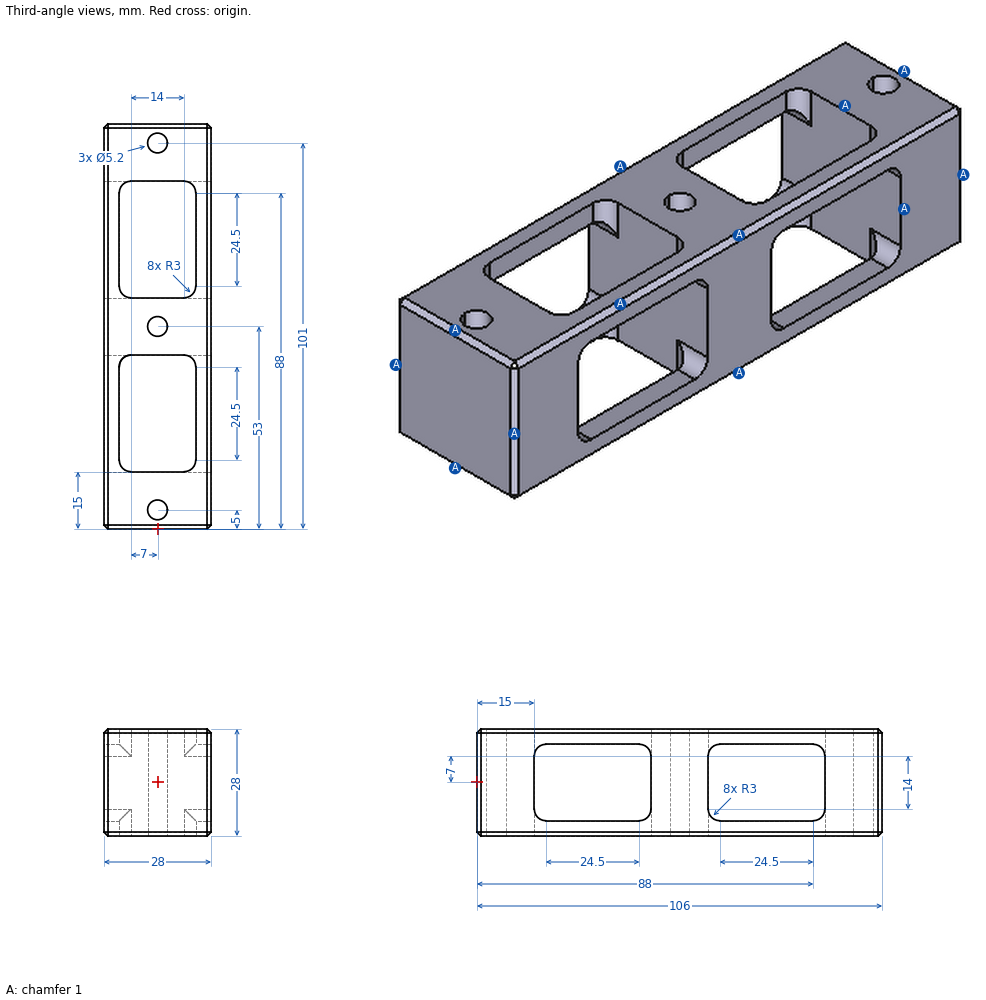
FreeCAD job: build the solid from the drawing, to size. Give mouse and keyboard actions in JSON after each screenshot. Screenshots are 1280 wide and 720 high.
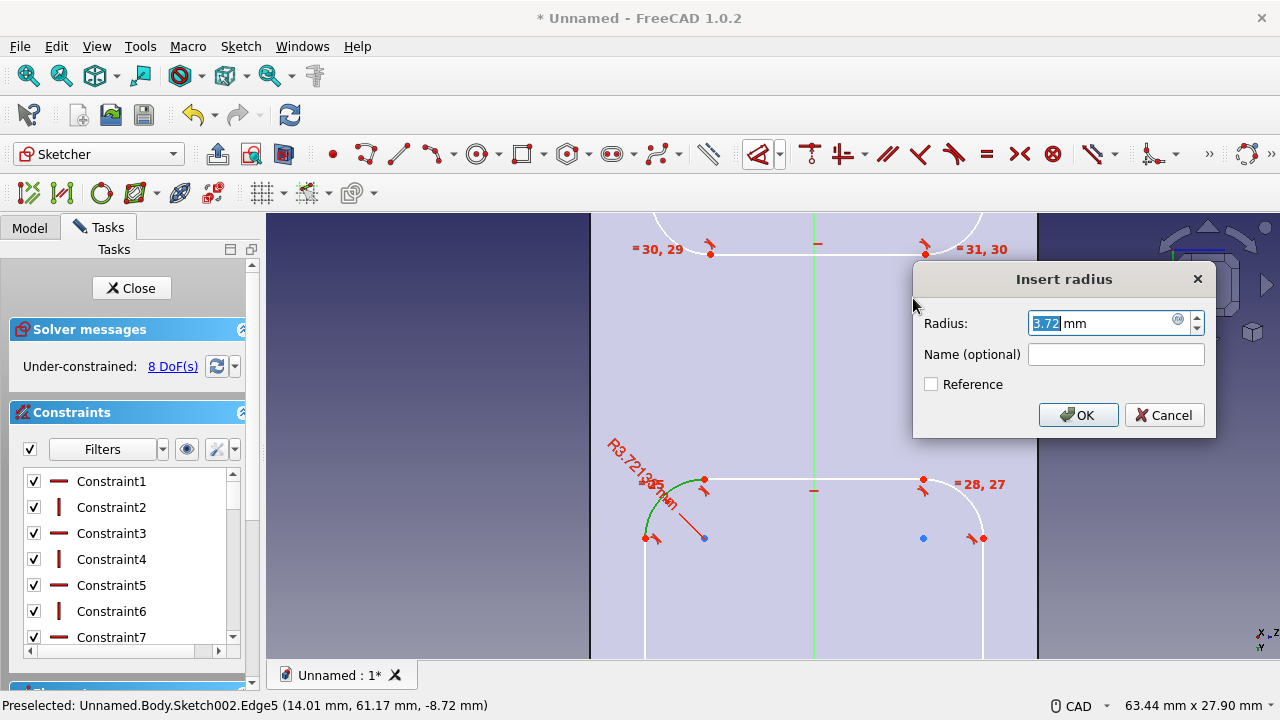
{"action": "type", "text": "3"}
{"action": "key", "text": "Return"}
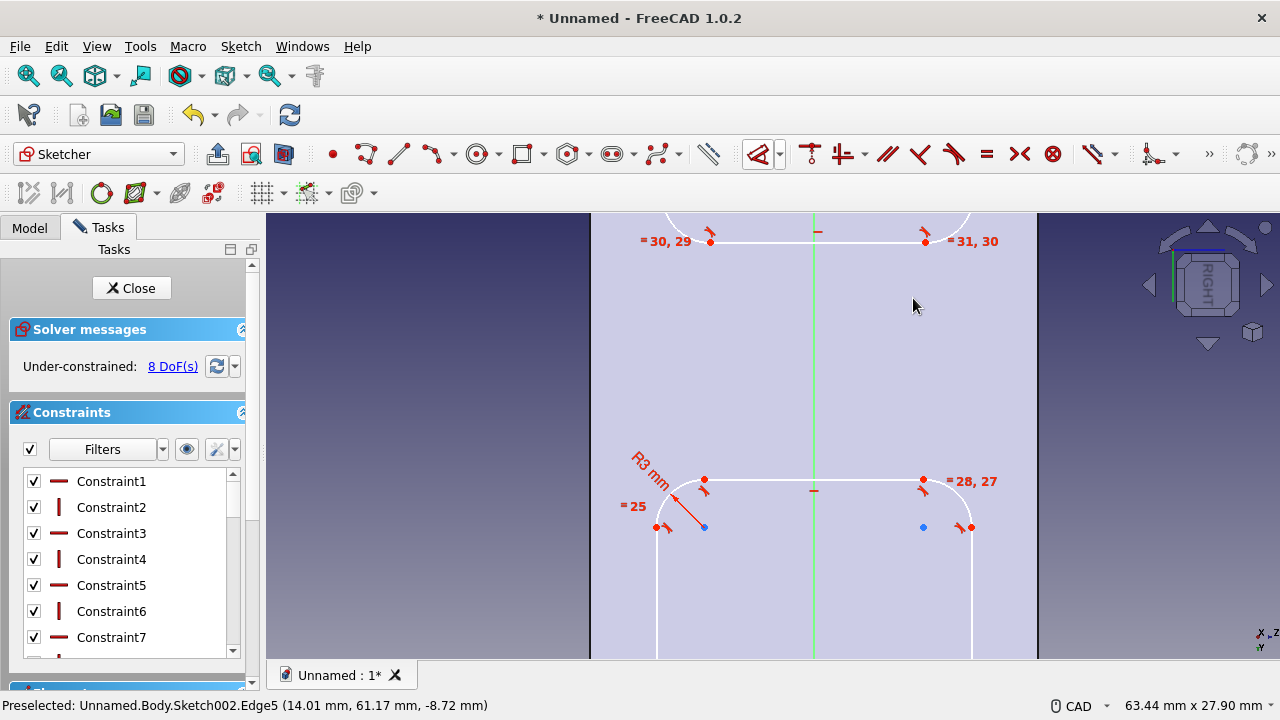
{"action": "scroll", "coordinate": [677, 486], "scroll_direction": "down", "scroll_amount": 8}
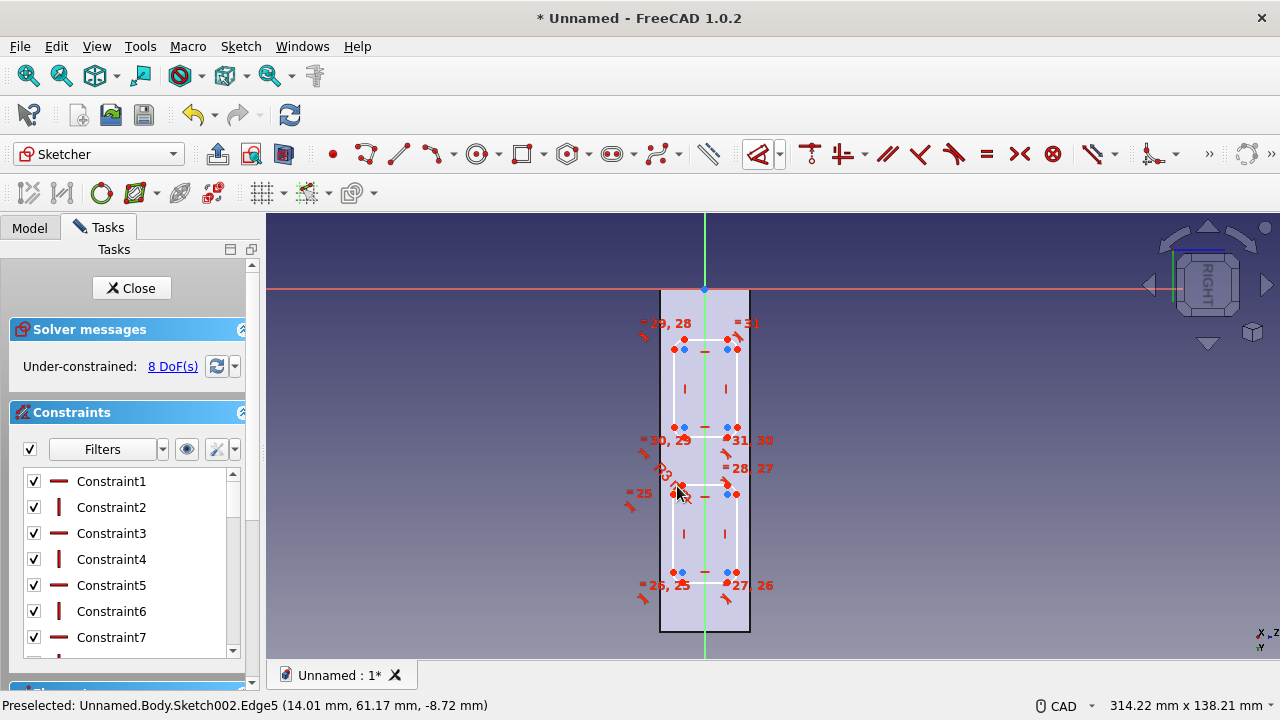
{"action": "scroll", "coordinate": [714, 485], "scroll_direction": "up", "scroll_amount": 3}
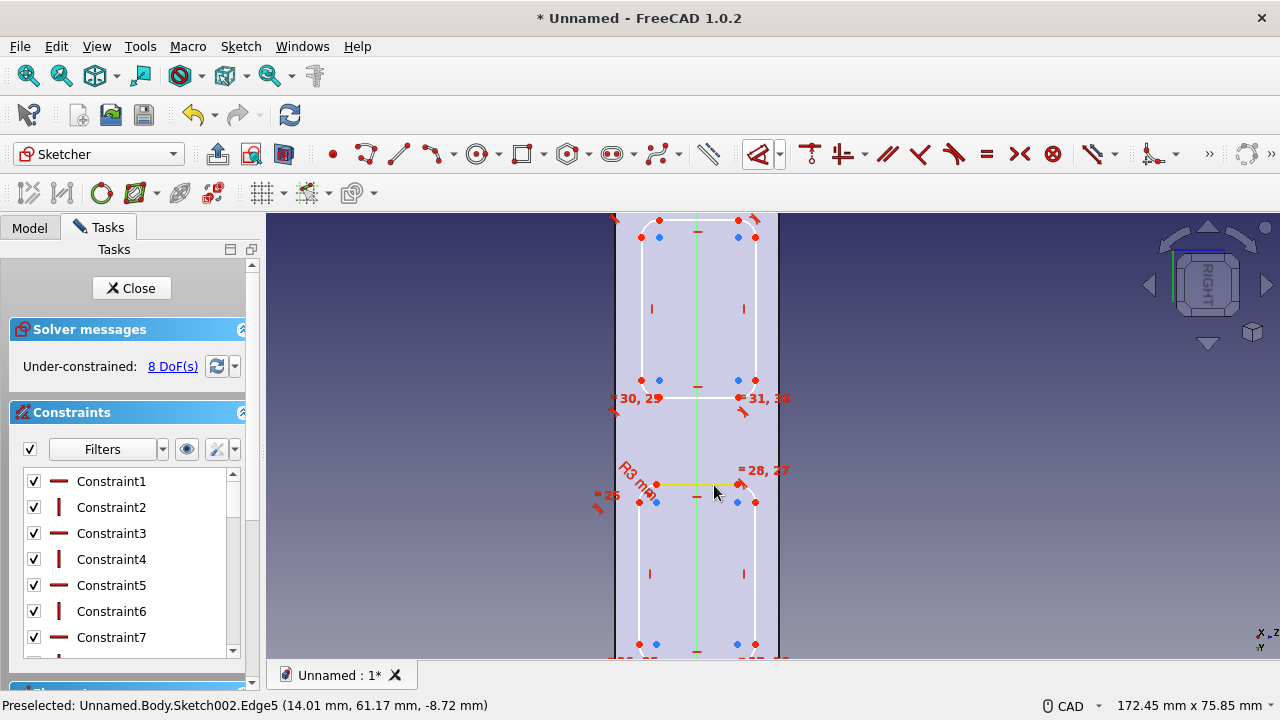
{"action": "left_click", "coordinate": [713, 485]}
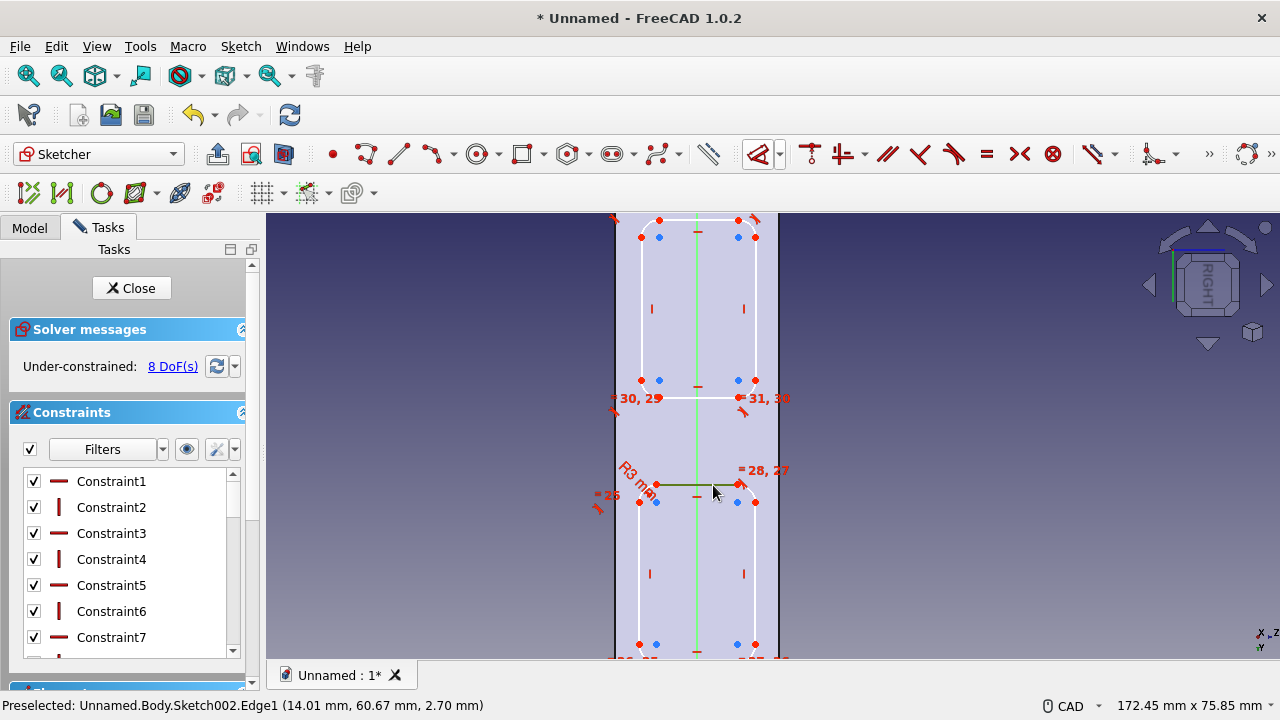
{"action": "left_click", "coordinate": [780, 154]}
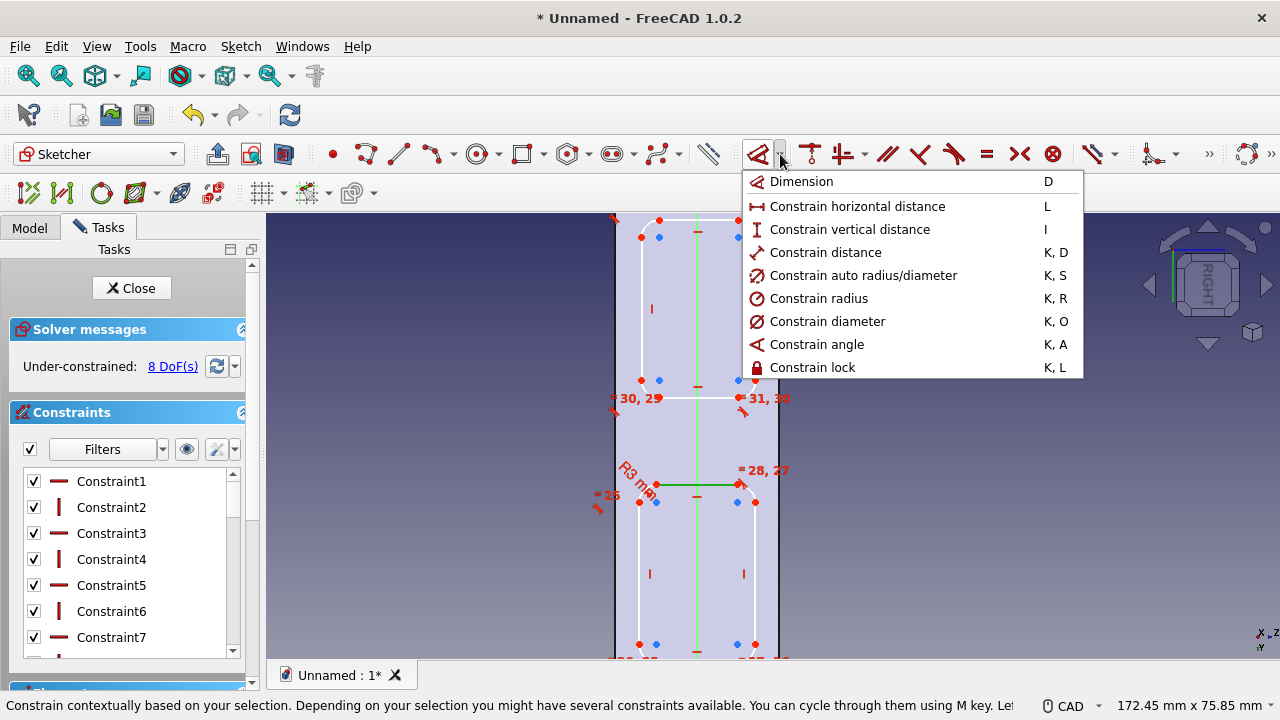
{"action": "left_click", "coordinate": [913, 206]}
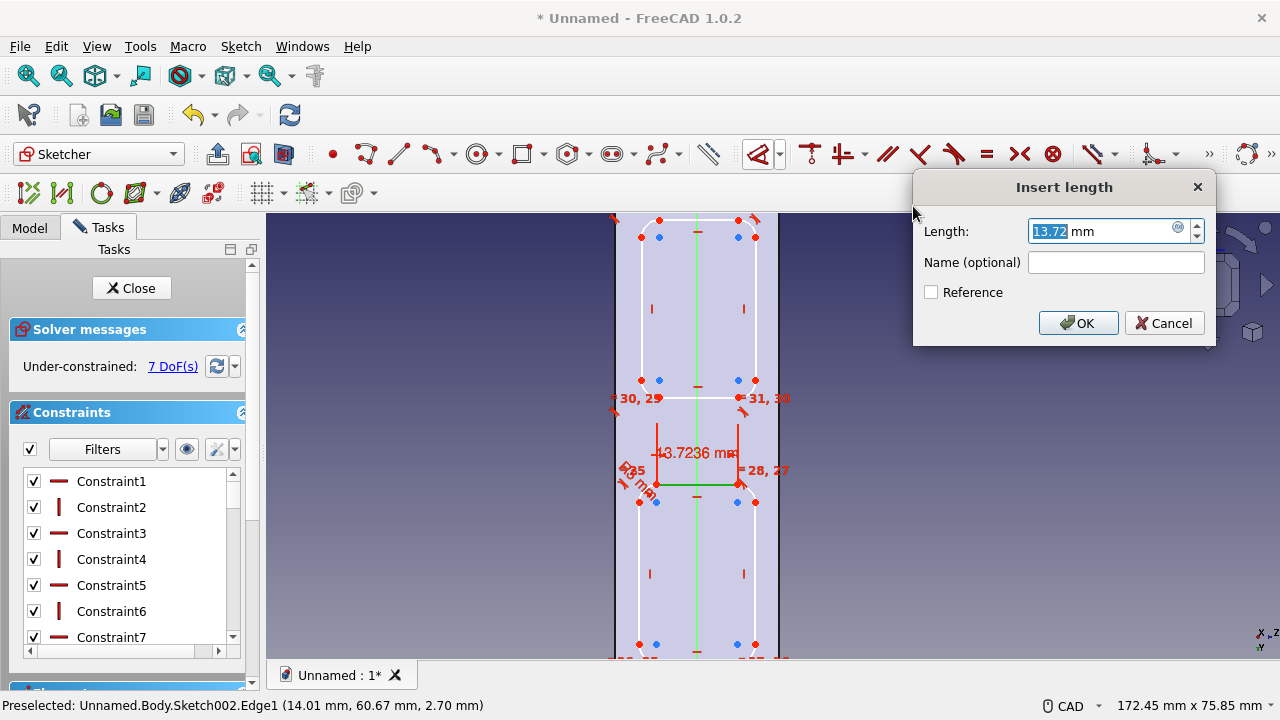
{"action": "type", "text": "14"}
{"action": "key", "text": "Return"}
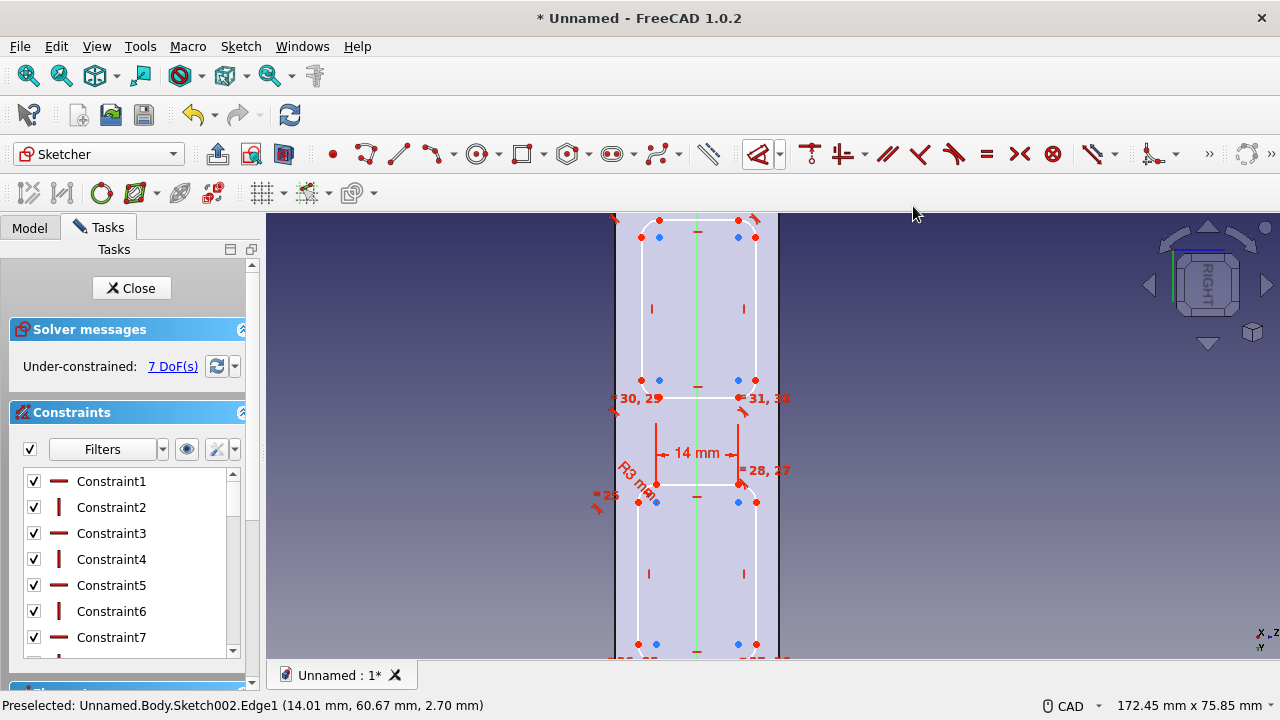
{"action": "scroll", "coordinate": [713, 485], "scroll_direction": "down", "scroll_amount": 3}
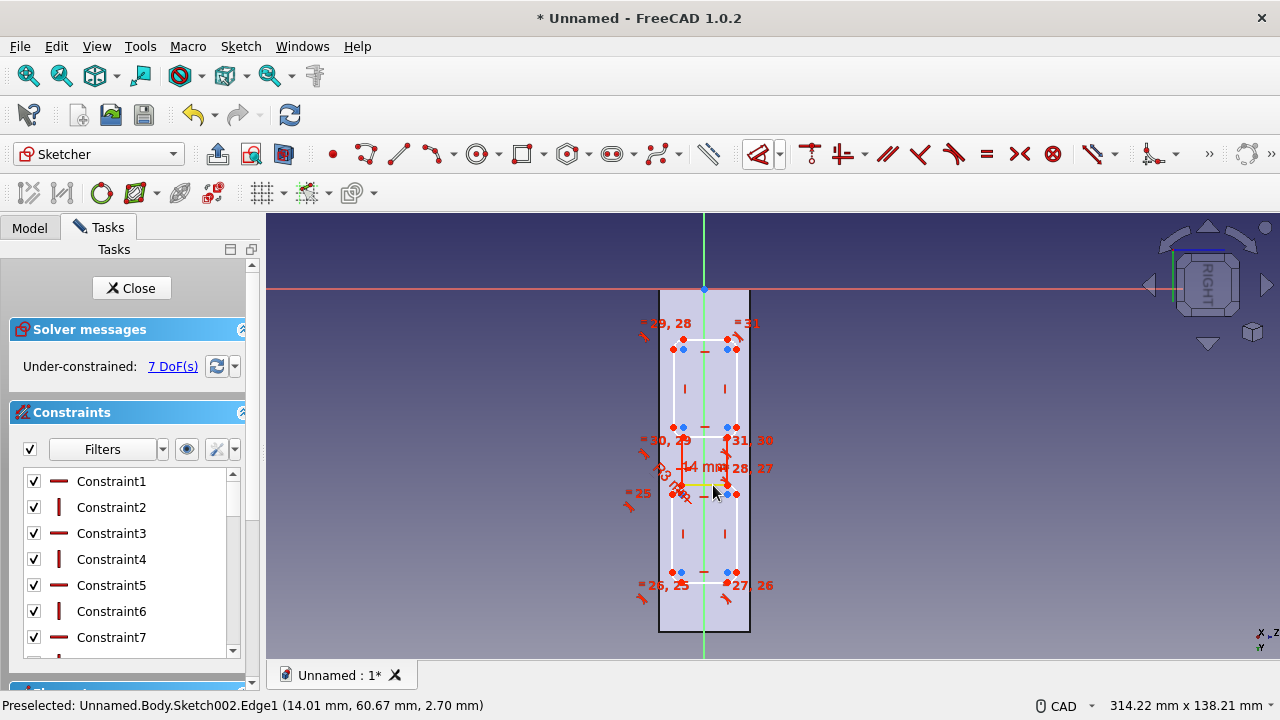
{"action": "scroll", "coordinate": [714, 340], "scroll_direction": "up", "scroll_amount": 2}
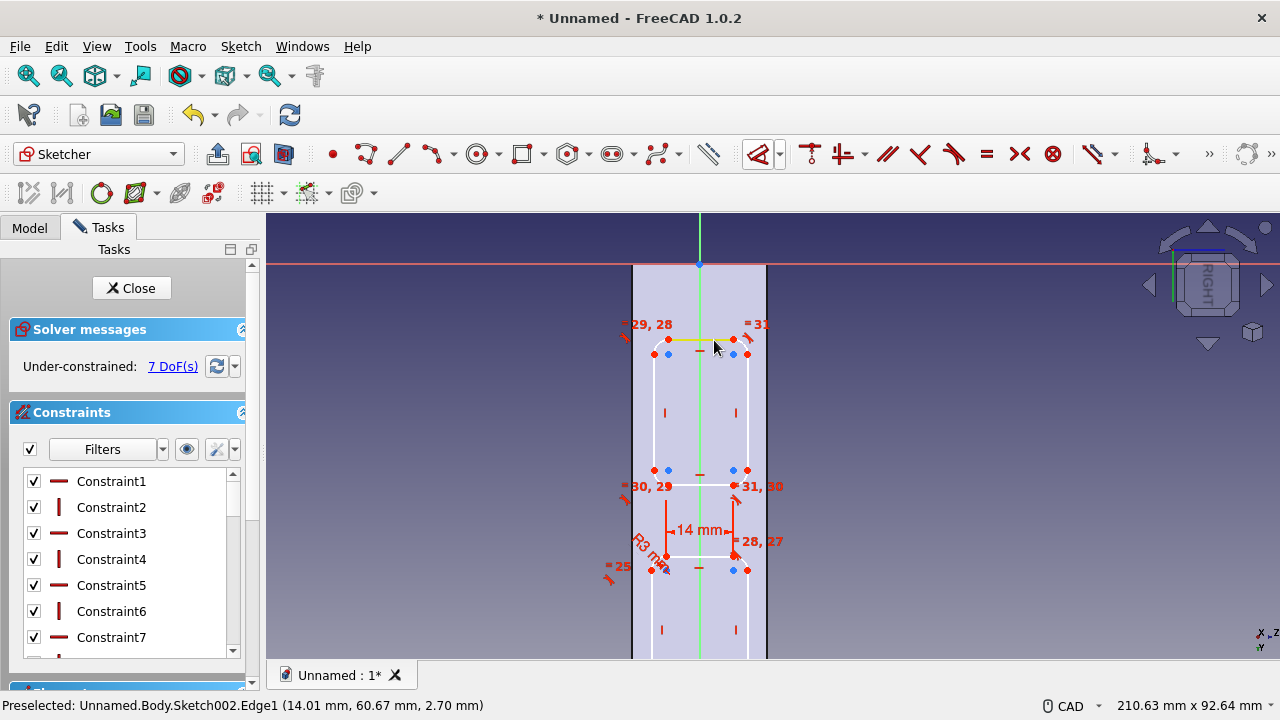
{"action": "left_click", "coordinate": [714, 340]}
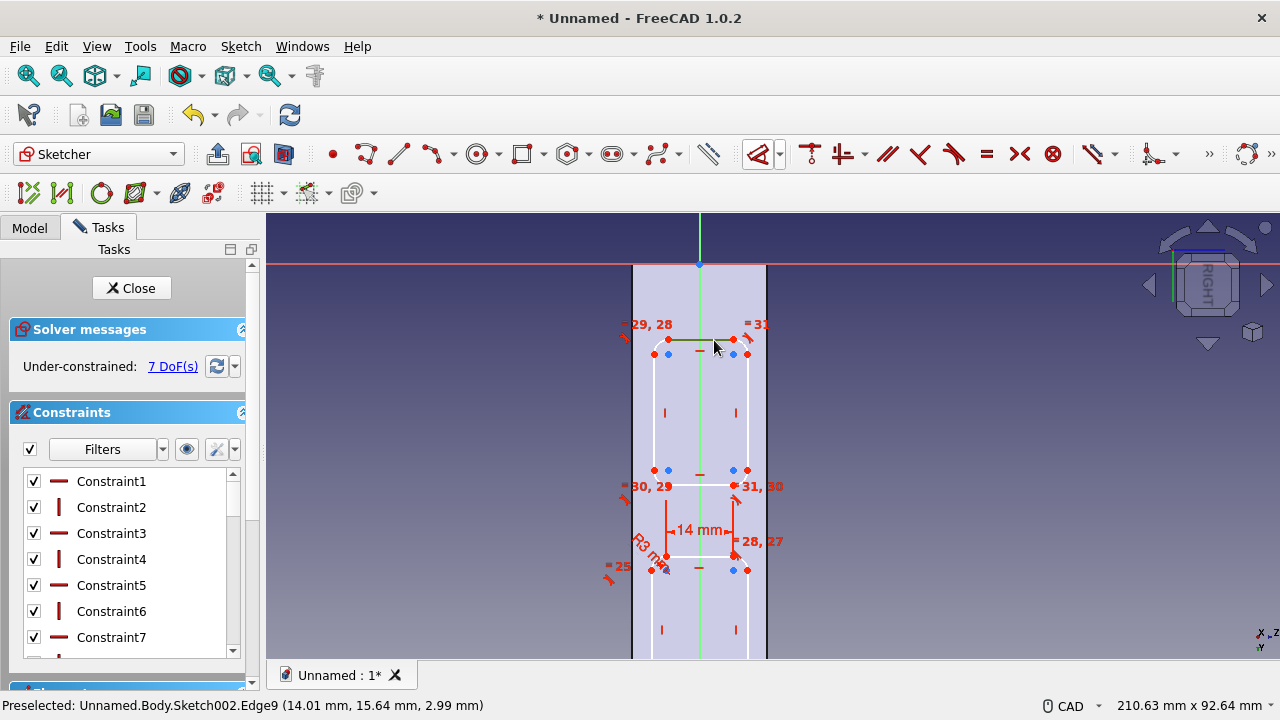
{"action": "left_click", "coordinate": [780, 154]}